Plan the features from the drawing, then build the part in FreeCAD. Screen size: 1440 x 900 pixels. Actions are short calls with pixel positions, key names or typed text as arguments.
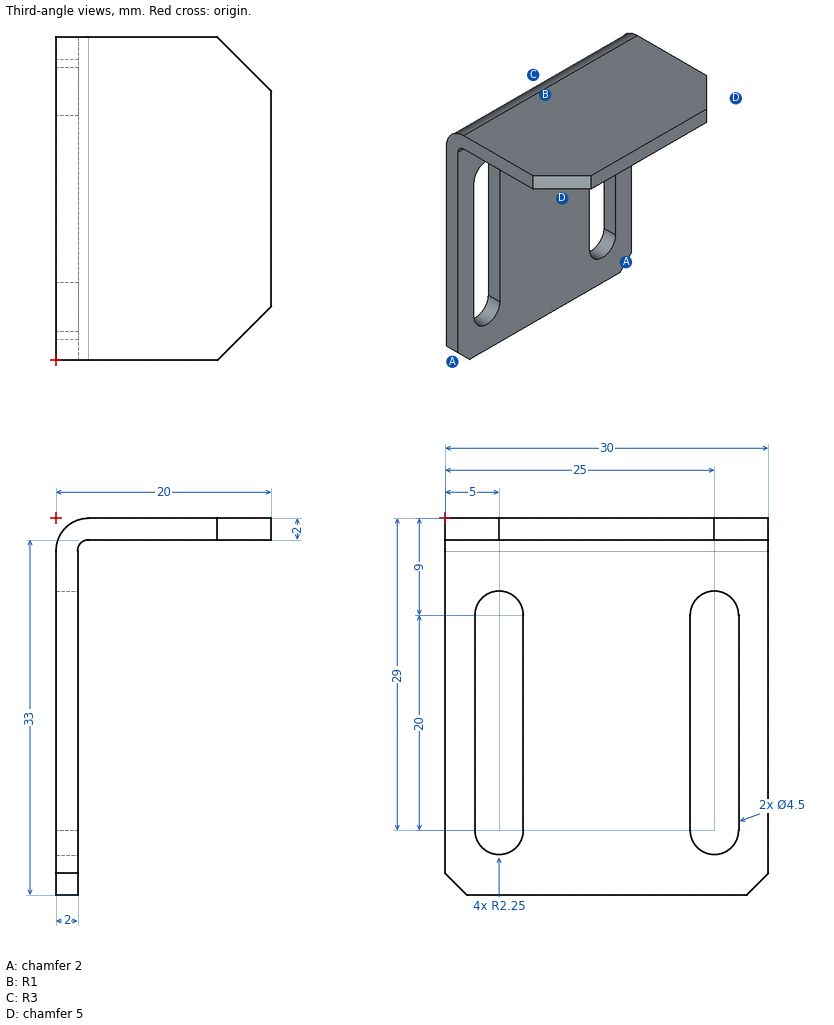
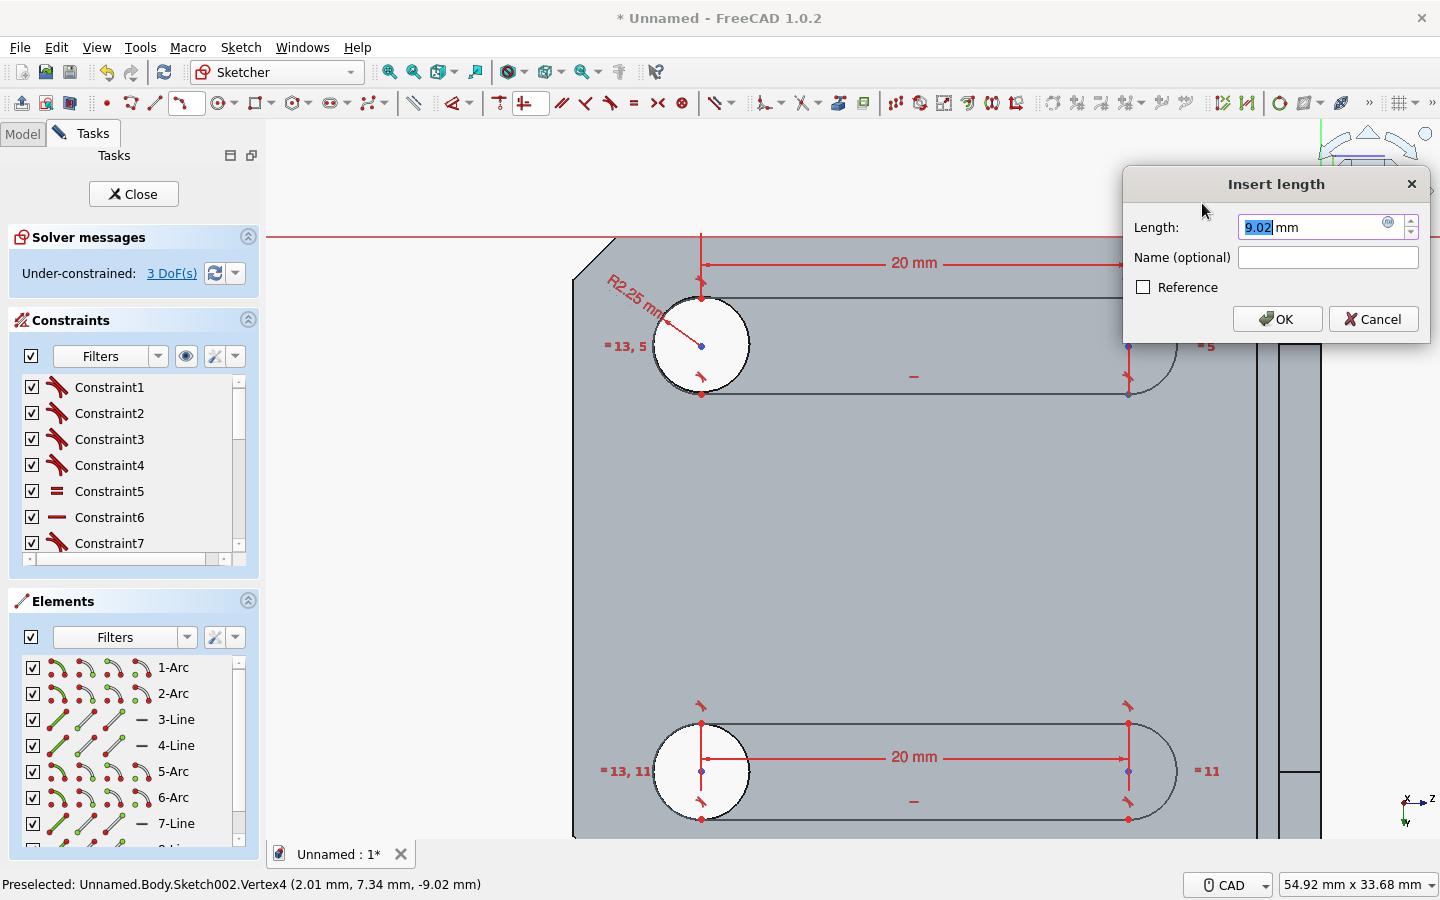
text(9)
key(Return)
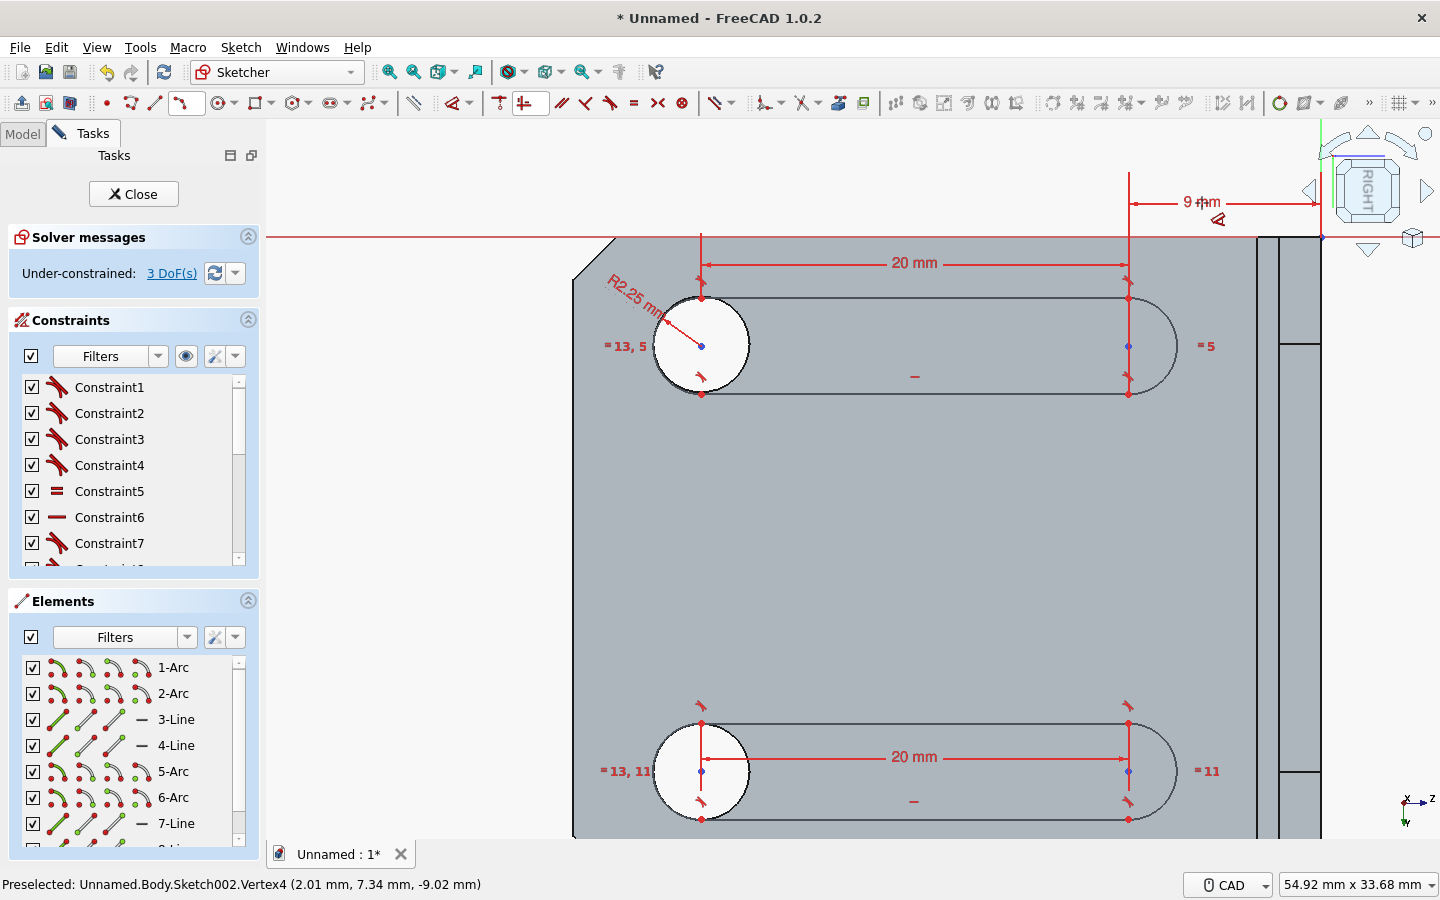
scroll(294, 255, down, 1)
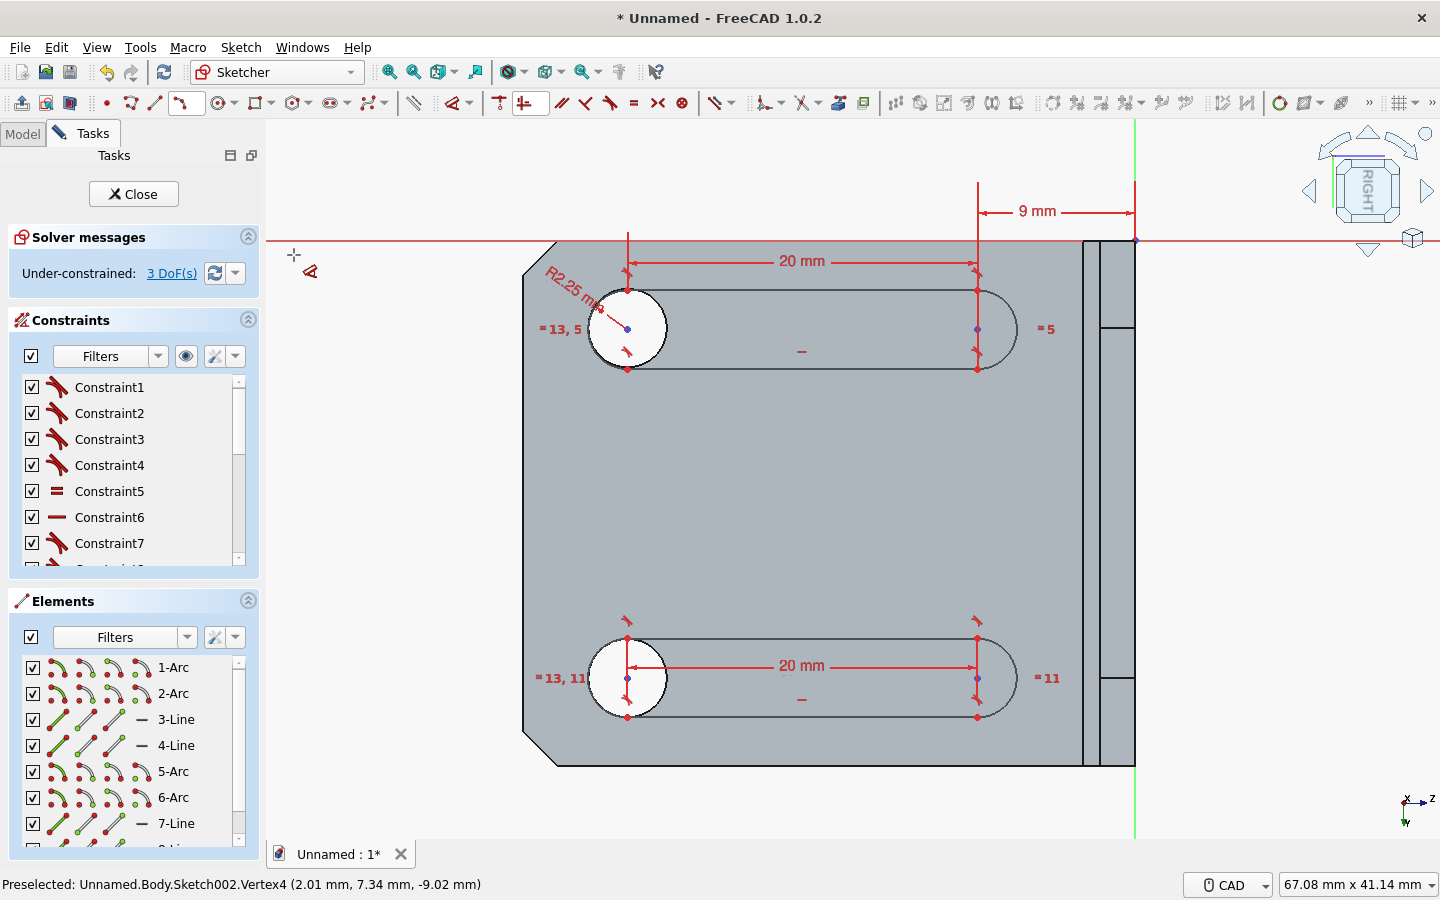
click(977, 717)
click(1111, 207)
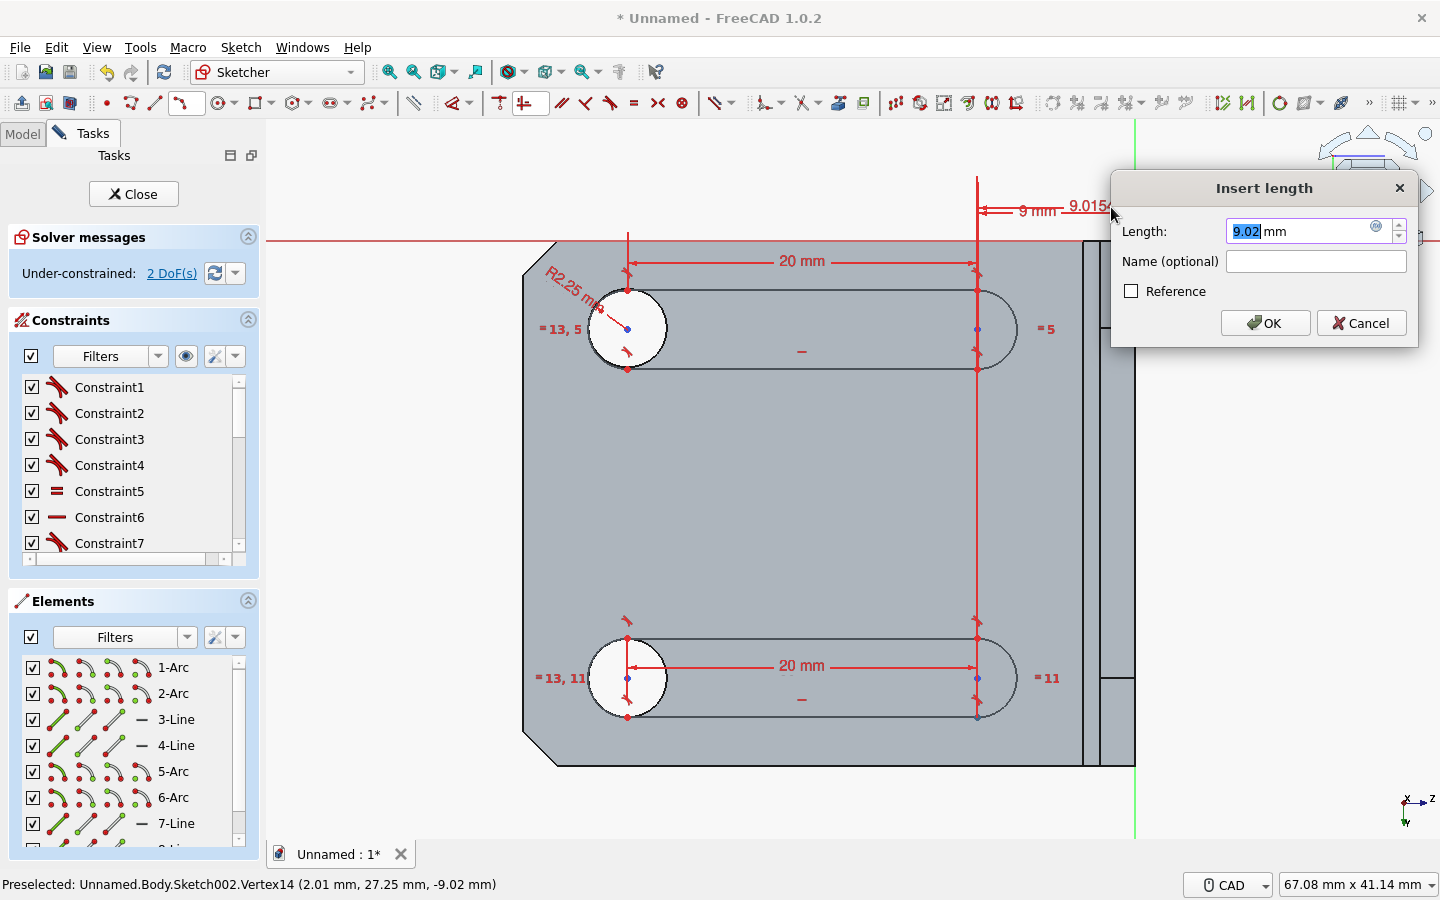
text(9)
key(Return)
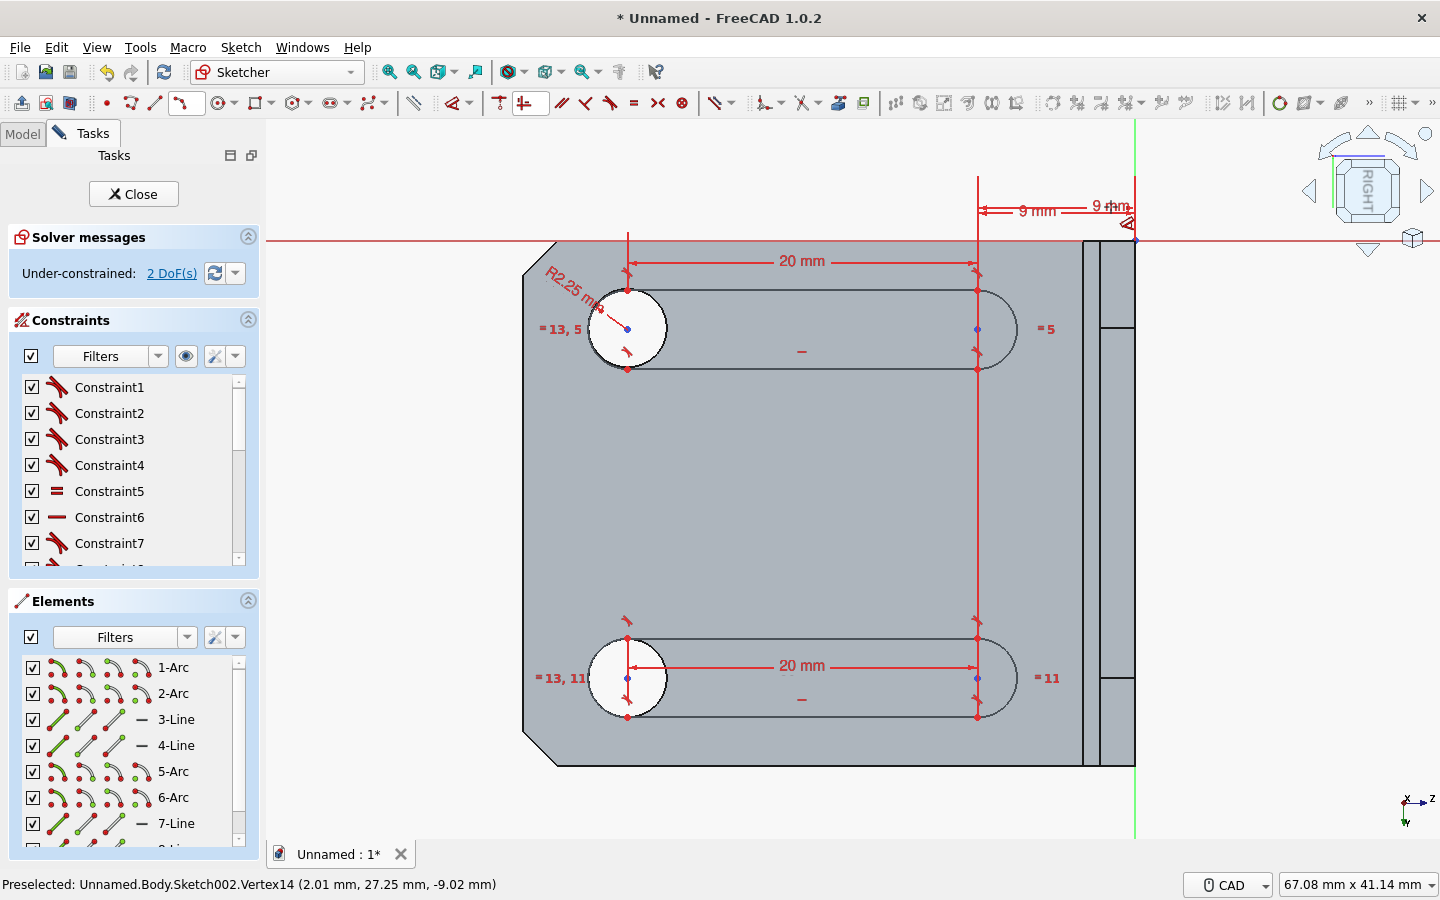
click(628, 330)
click(1169, 285)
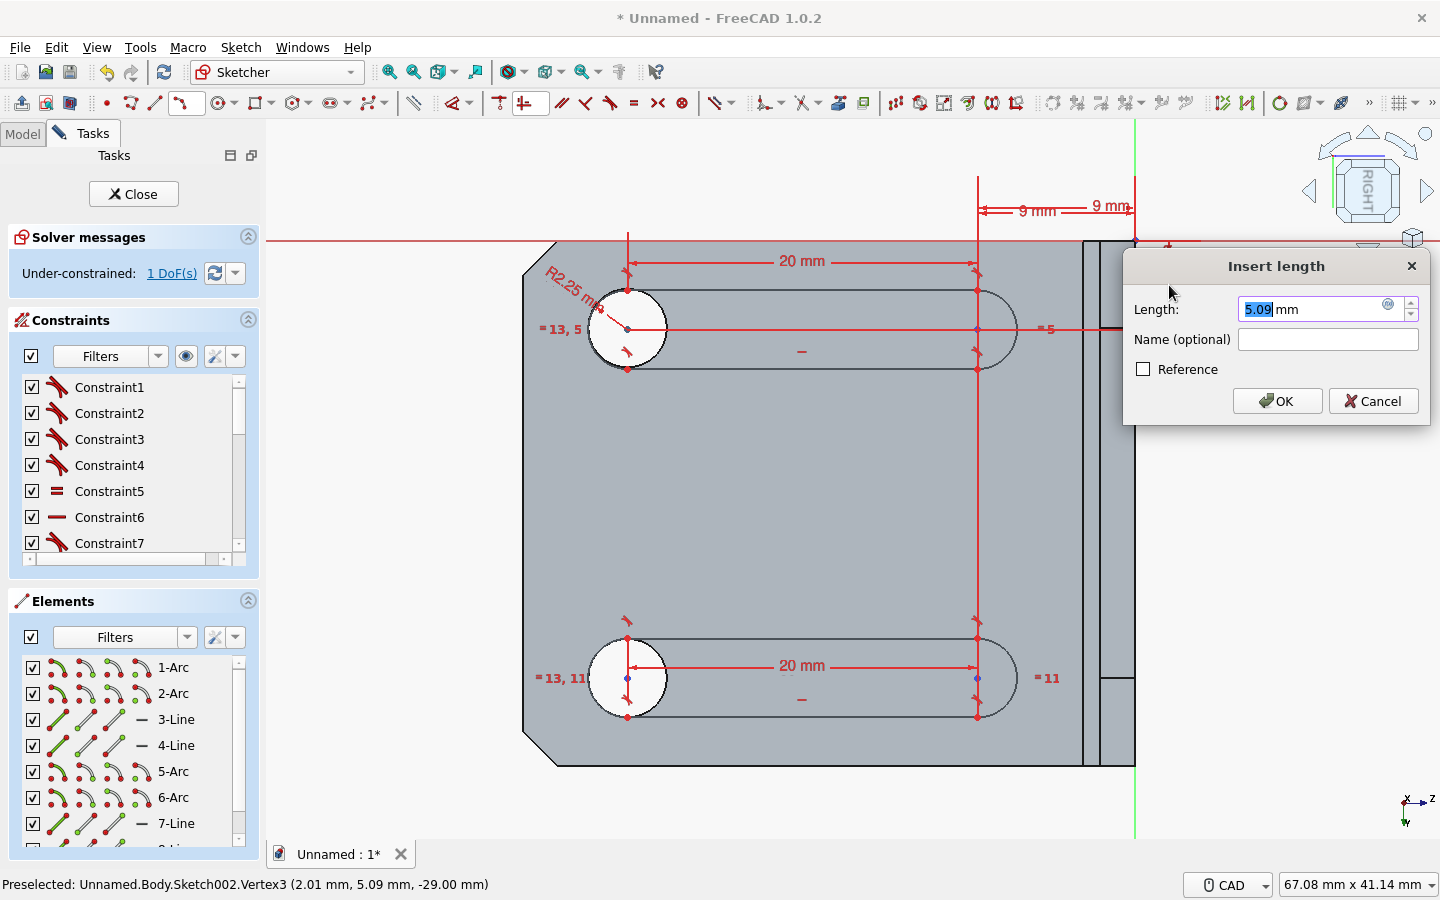
text(5)
key(Return)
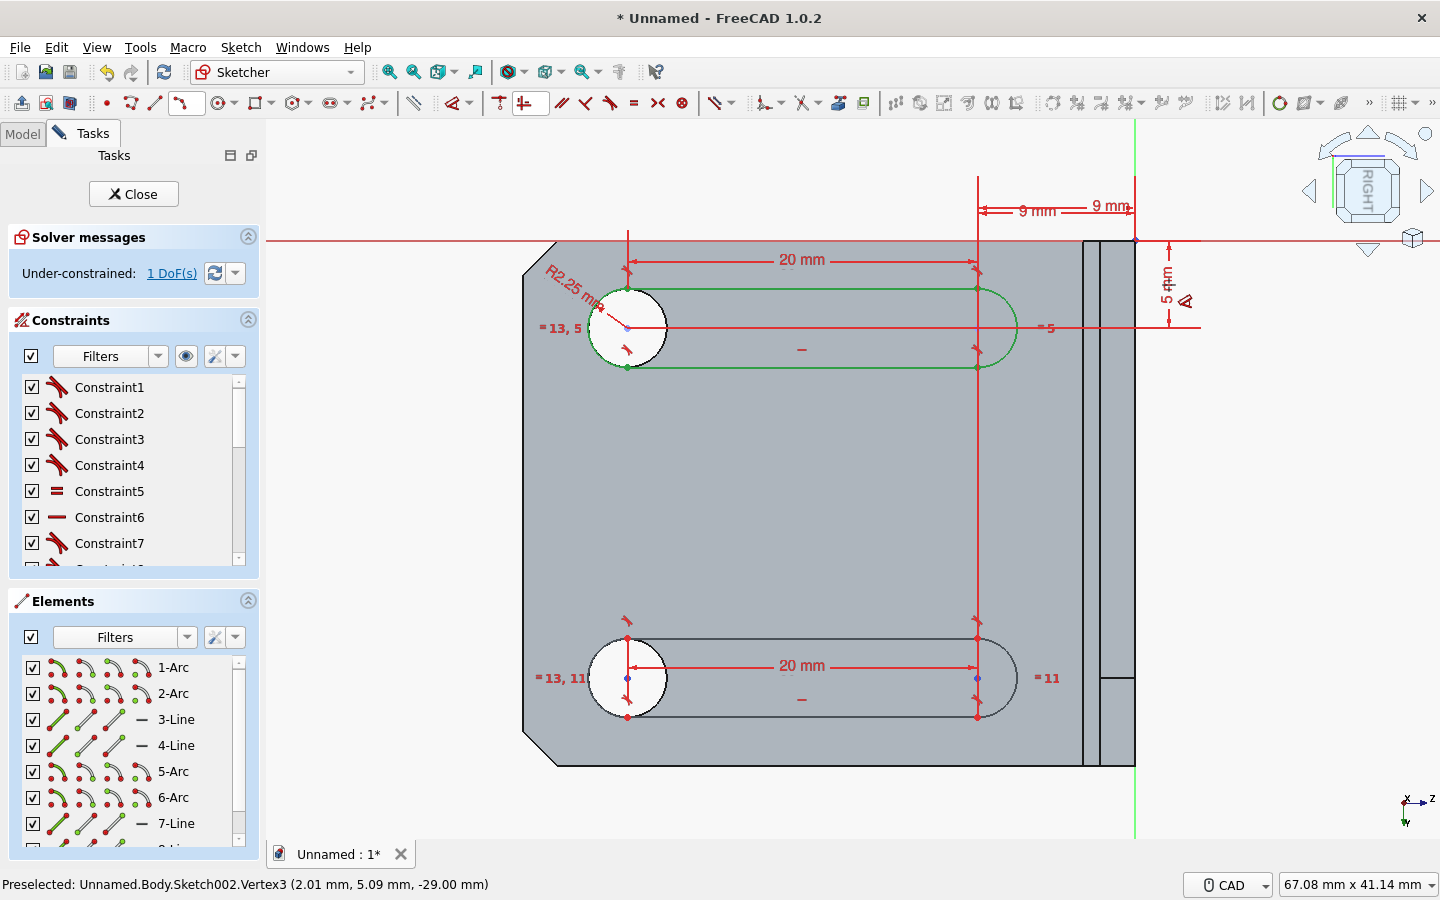
click(628, 678)
click(1169, 459)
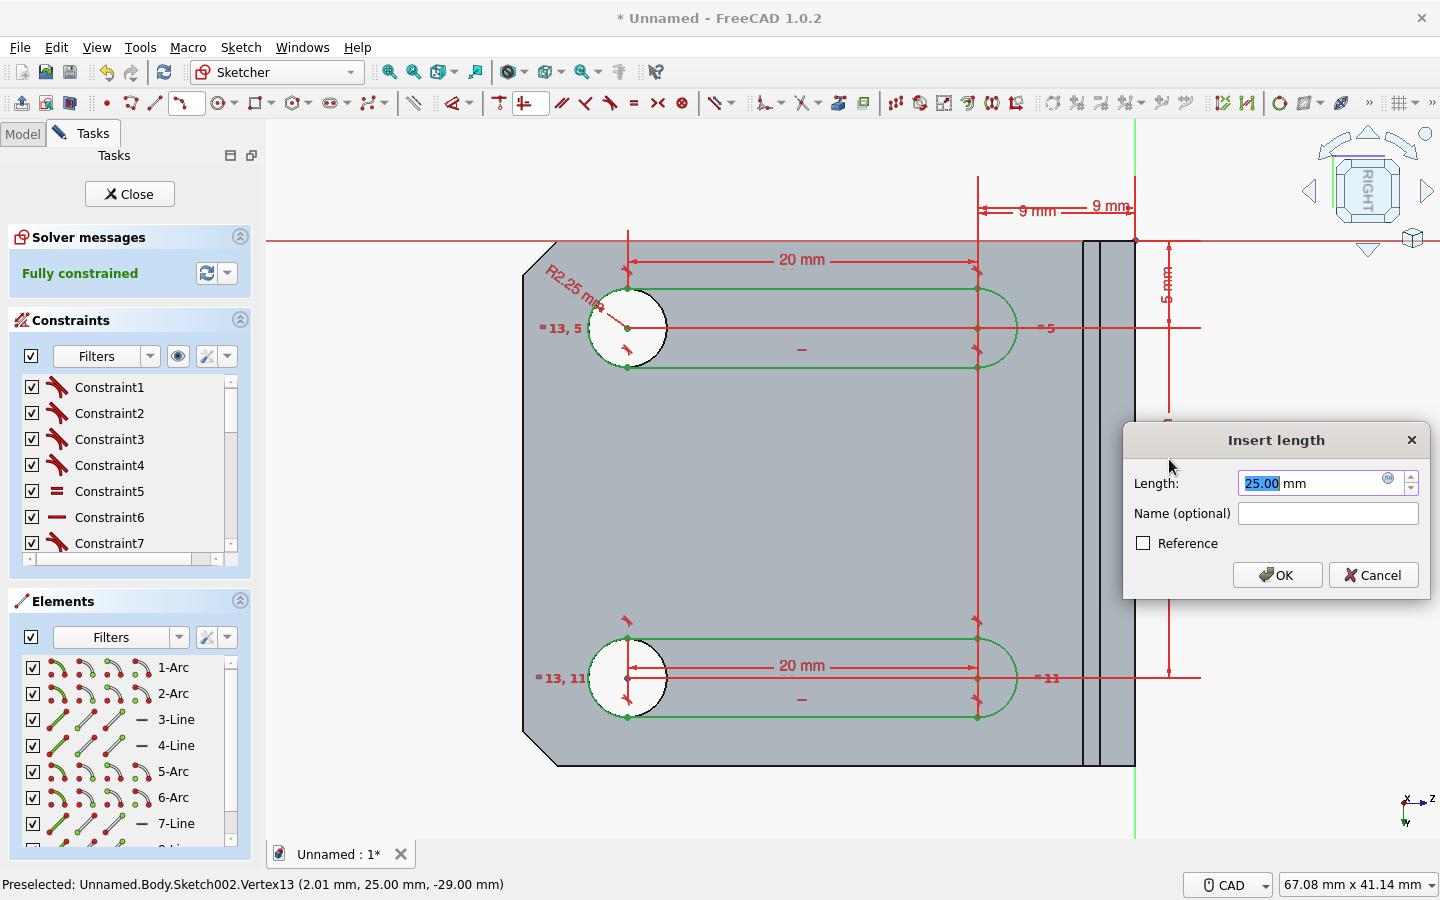
text(25)
key(Return)
key(Escape)